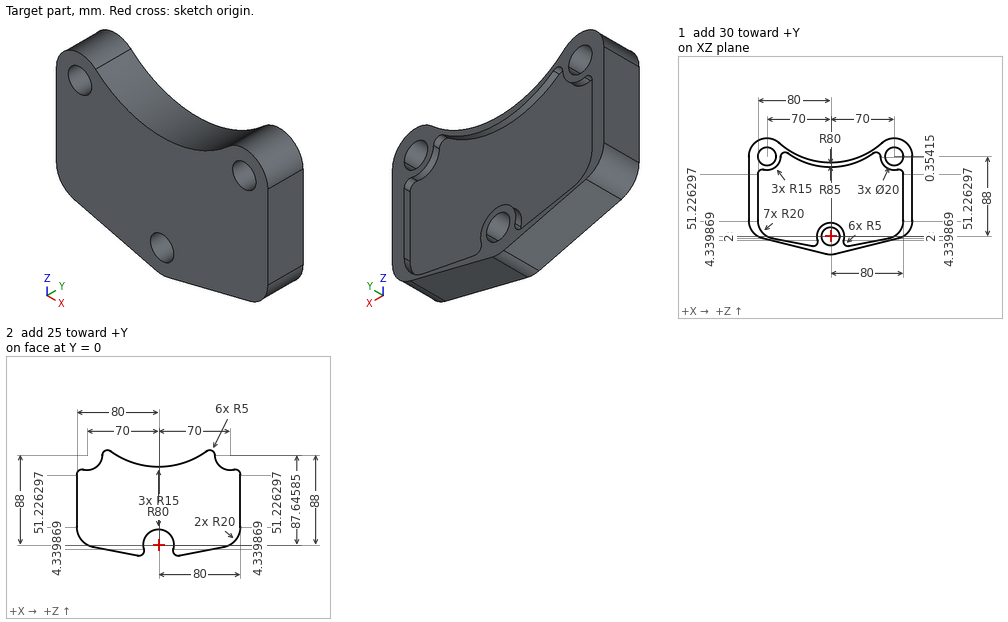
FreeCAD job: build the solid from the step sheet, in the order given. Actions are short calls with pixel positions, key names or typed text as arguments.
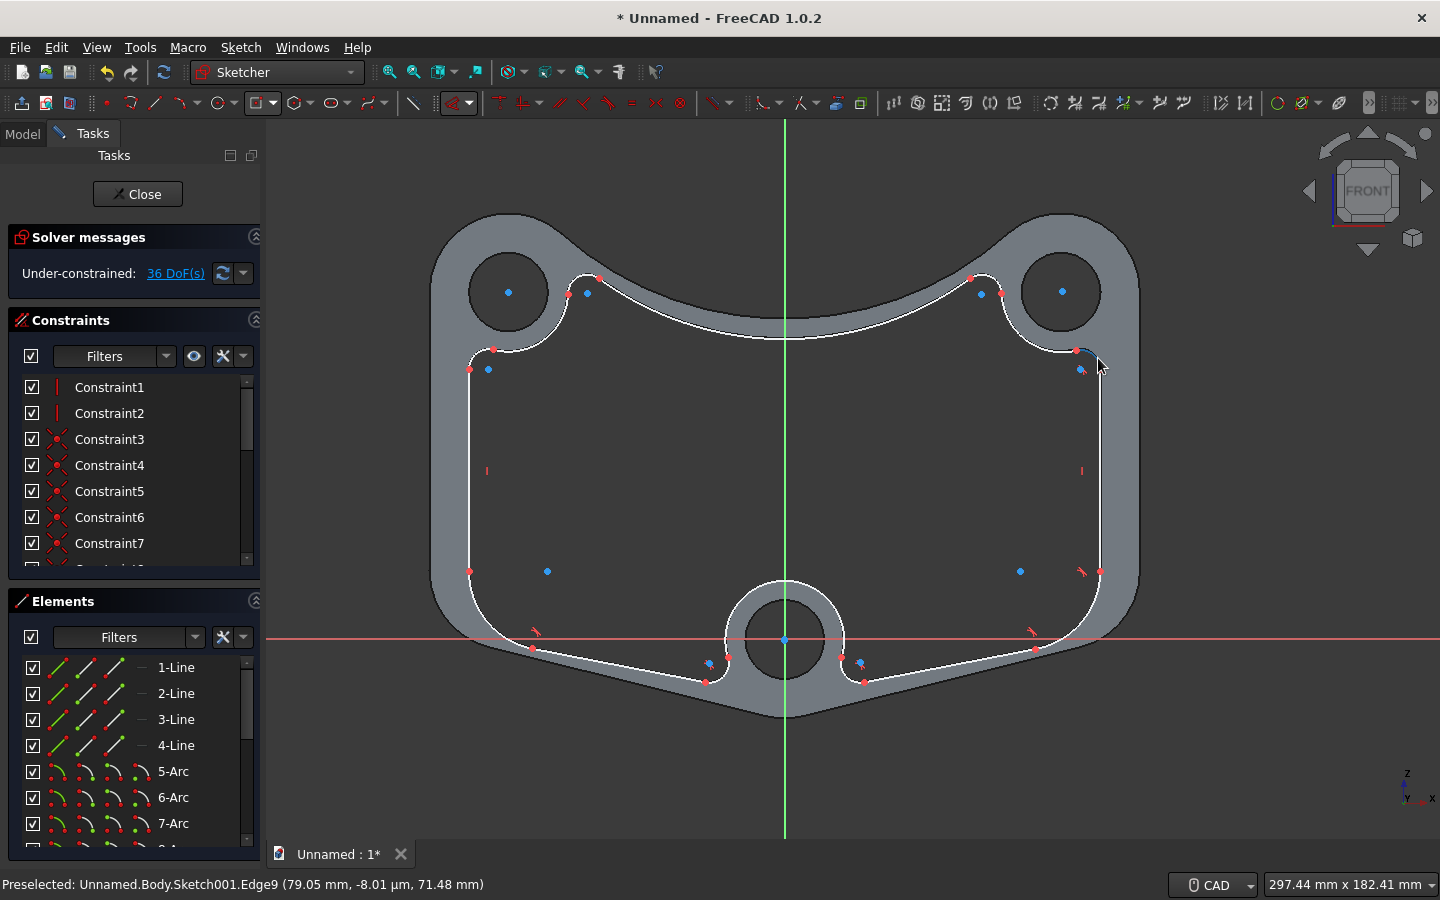
click(469, 430)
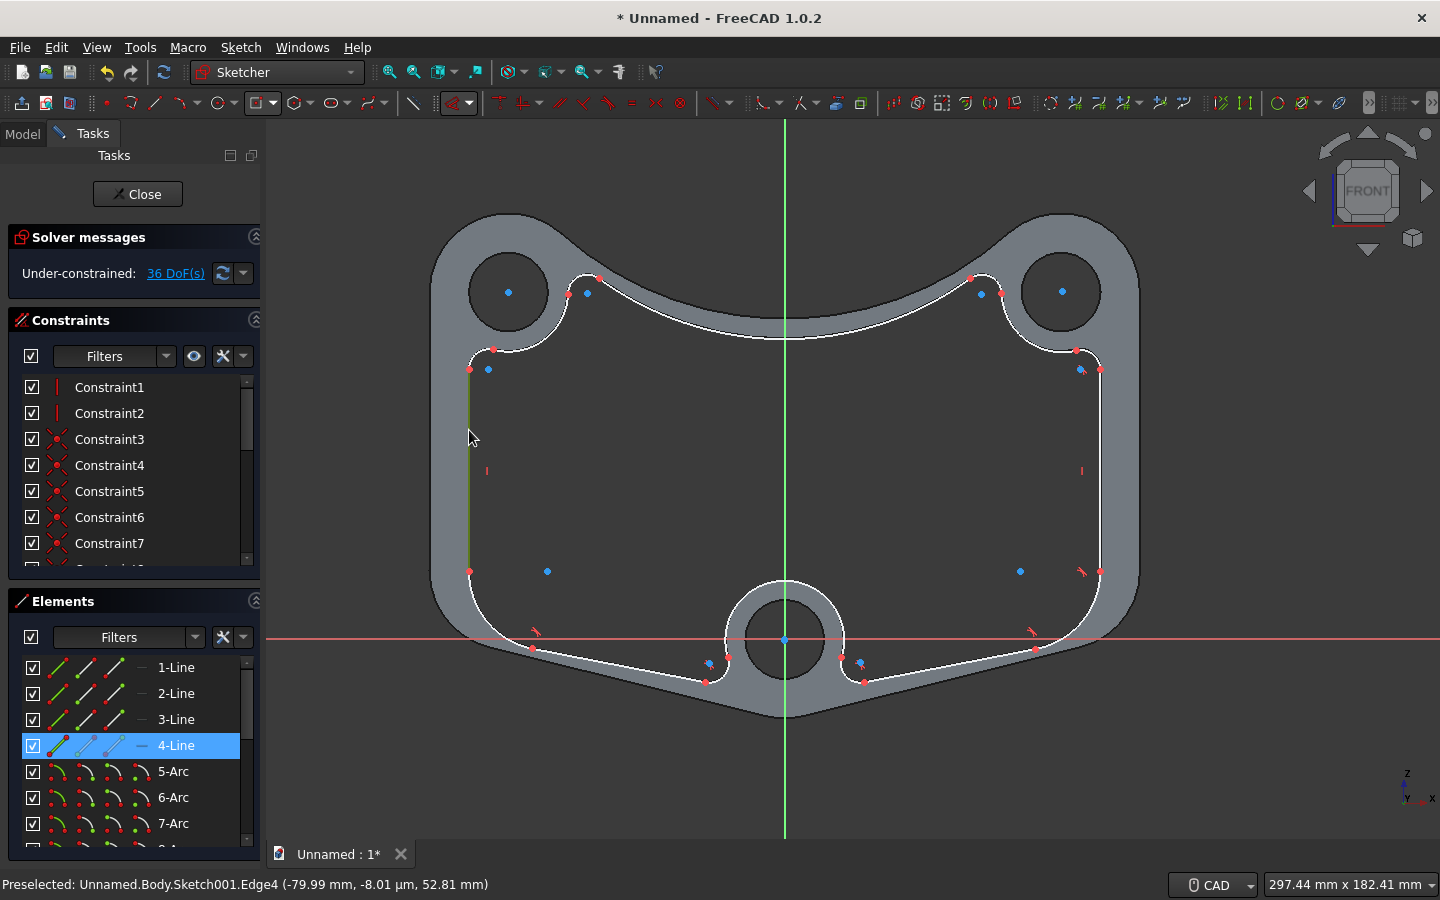
scroll(483, 350, up, 2)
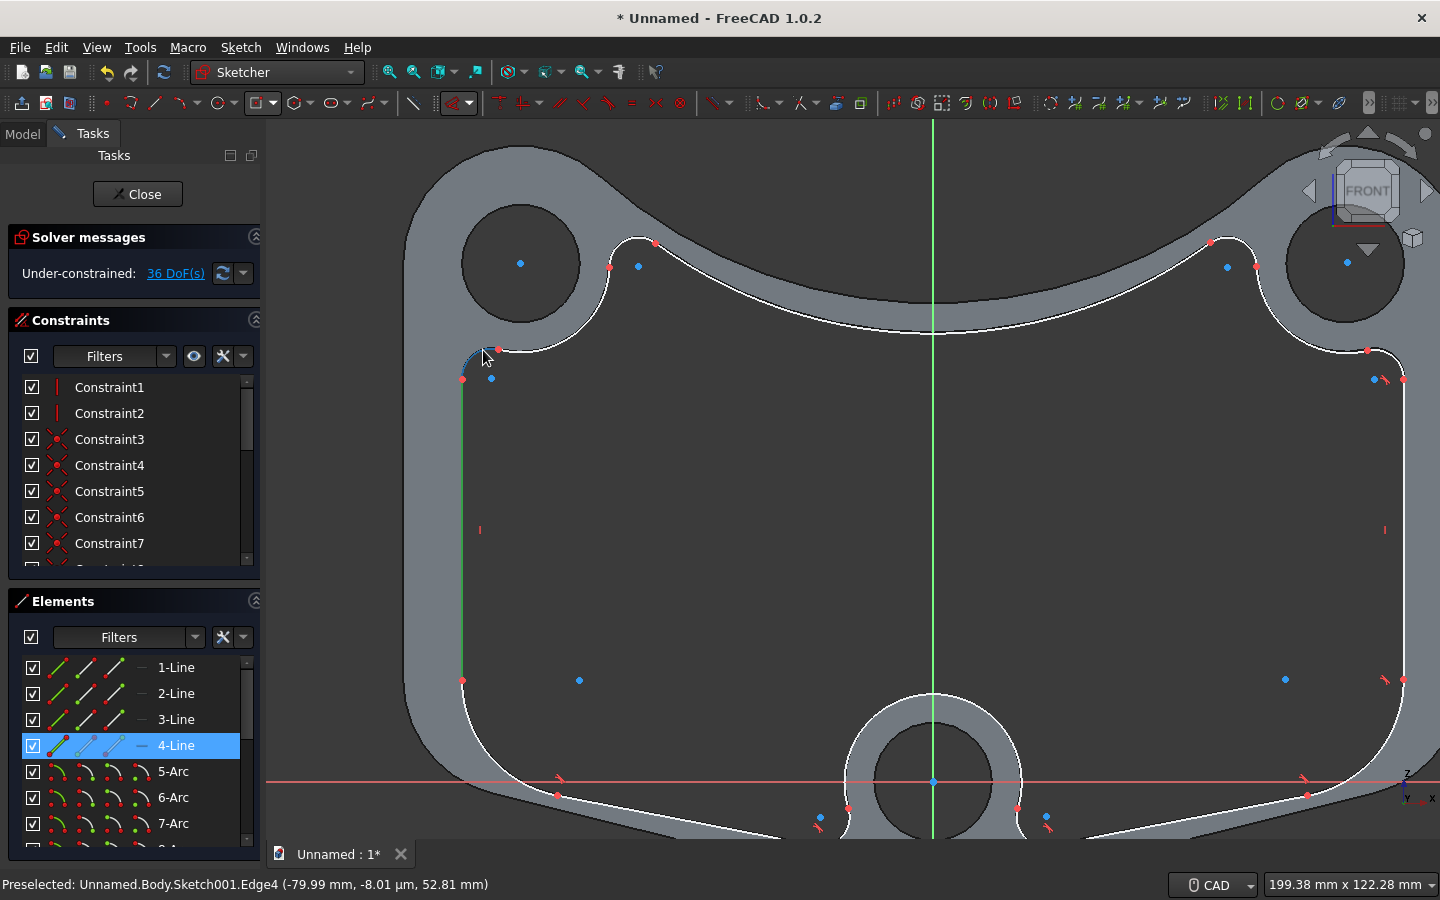
click(483, 350)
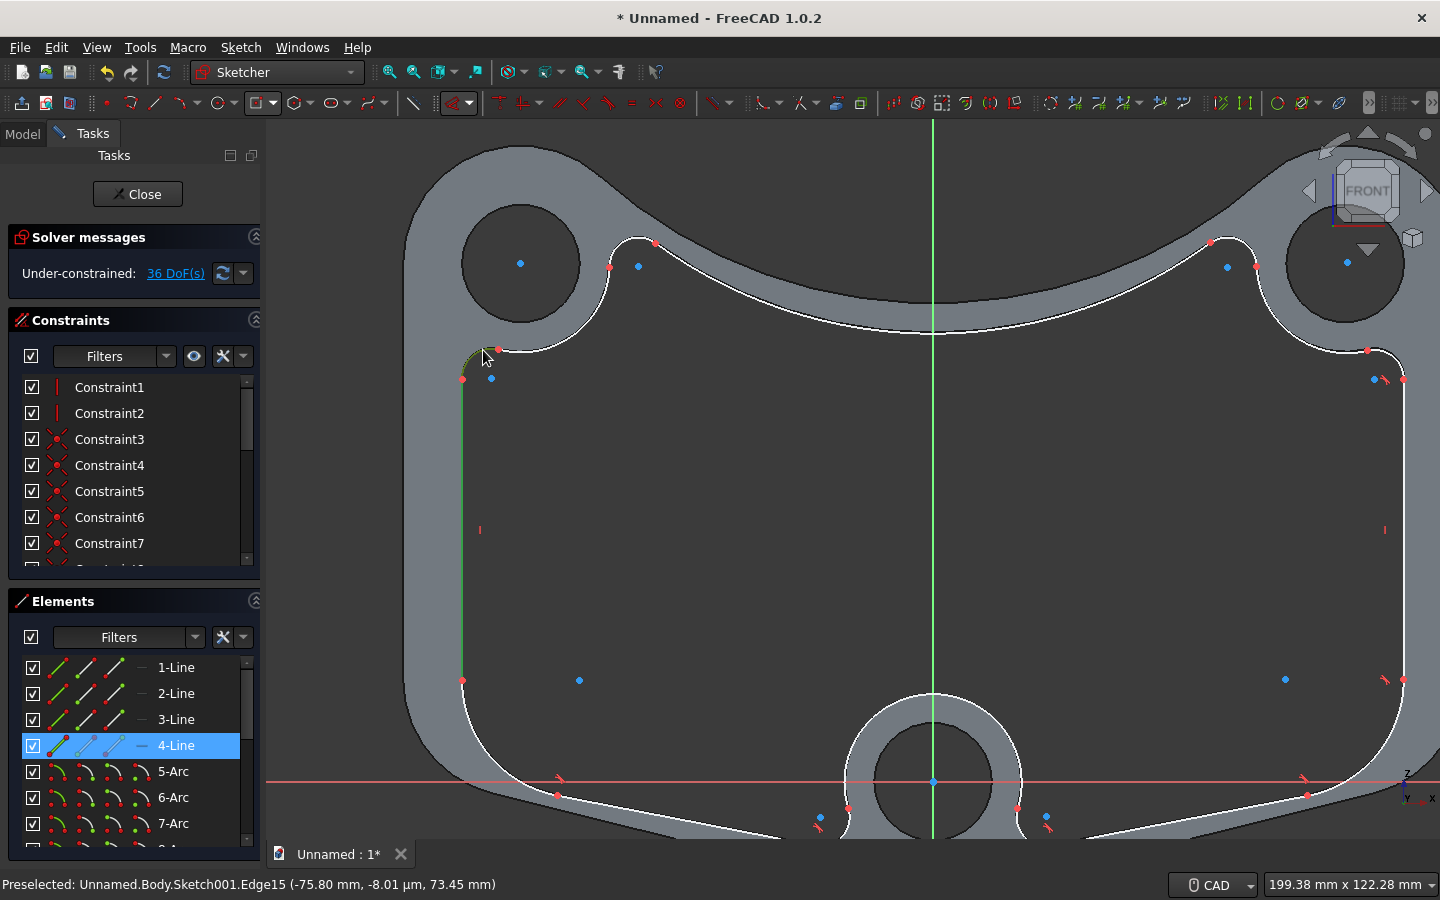
key(t)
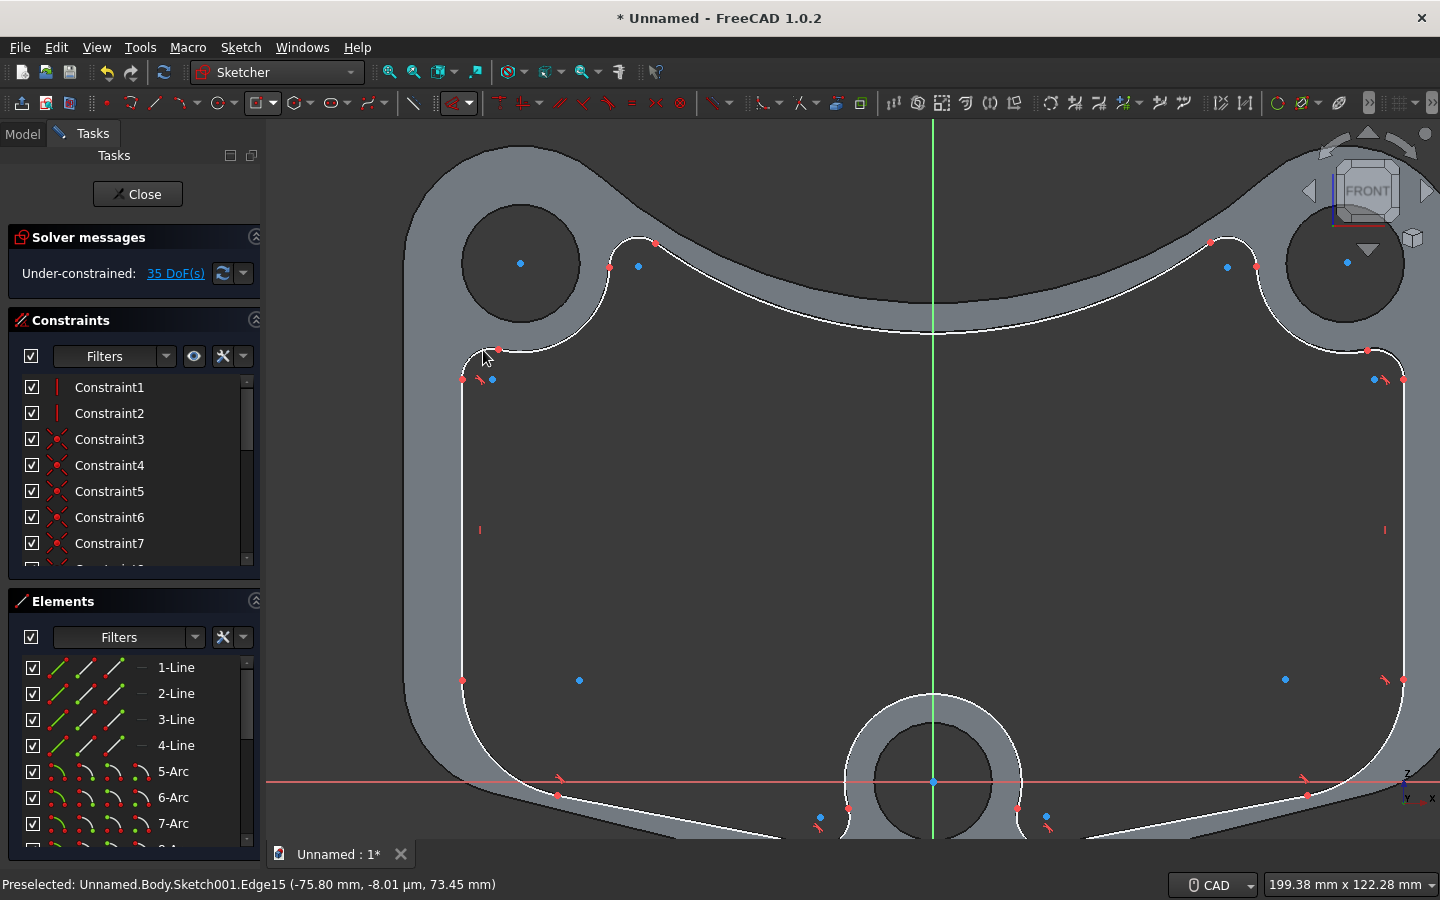
click(462, 470)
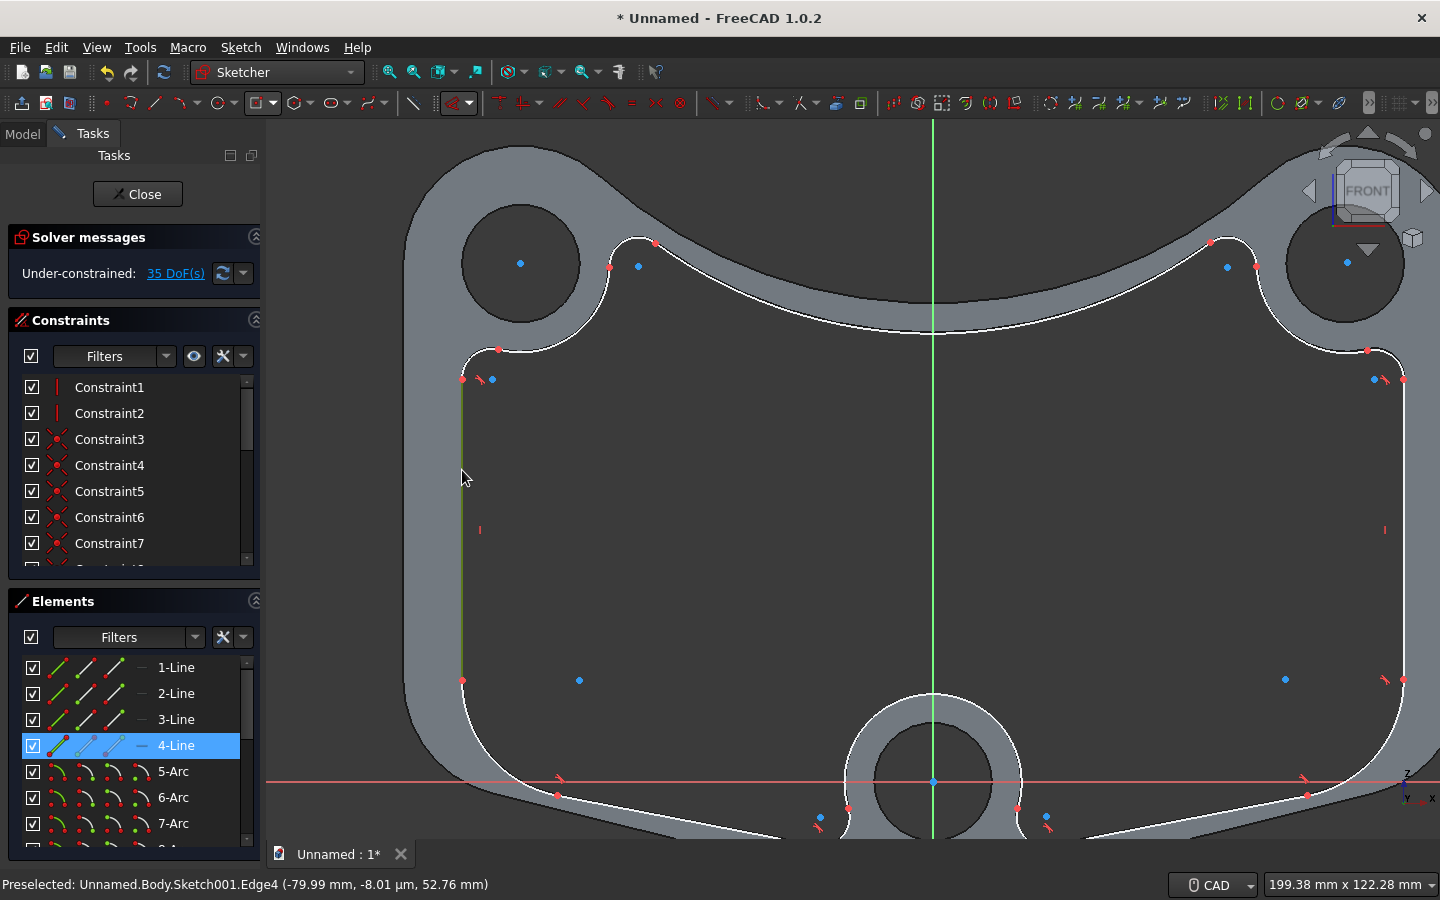
click(472, 728)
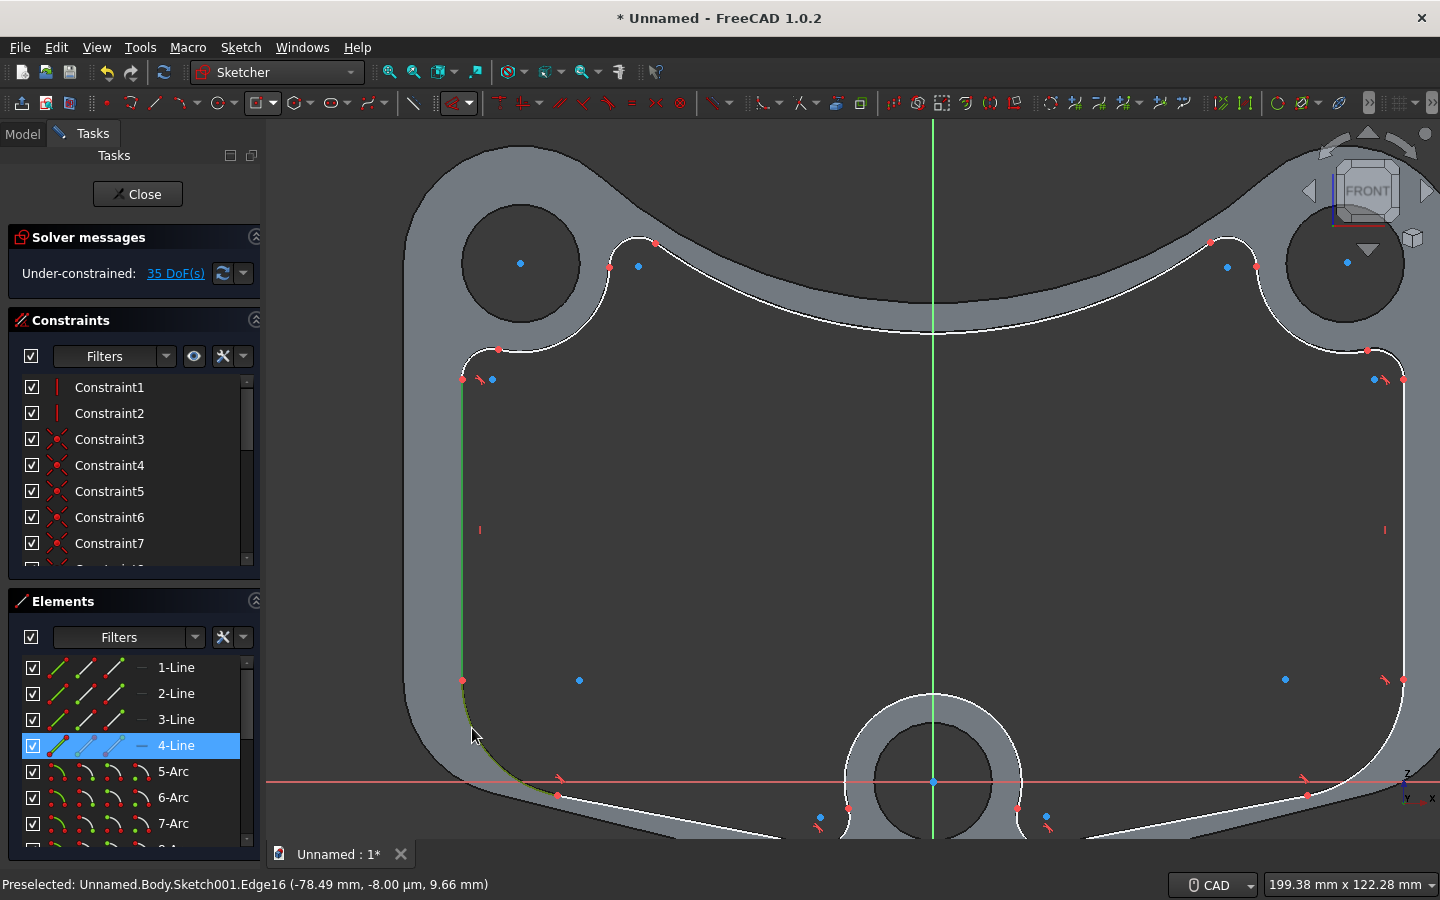
click(608, 104)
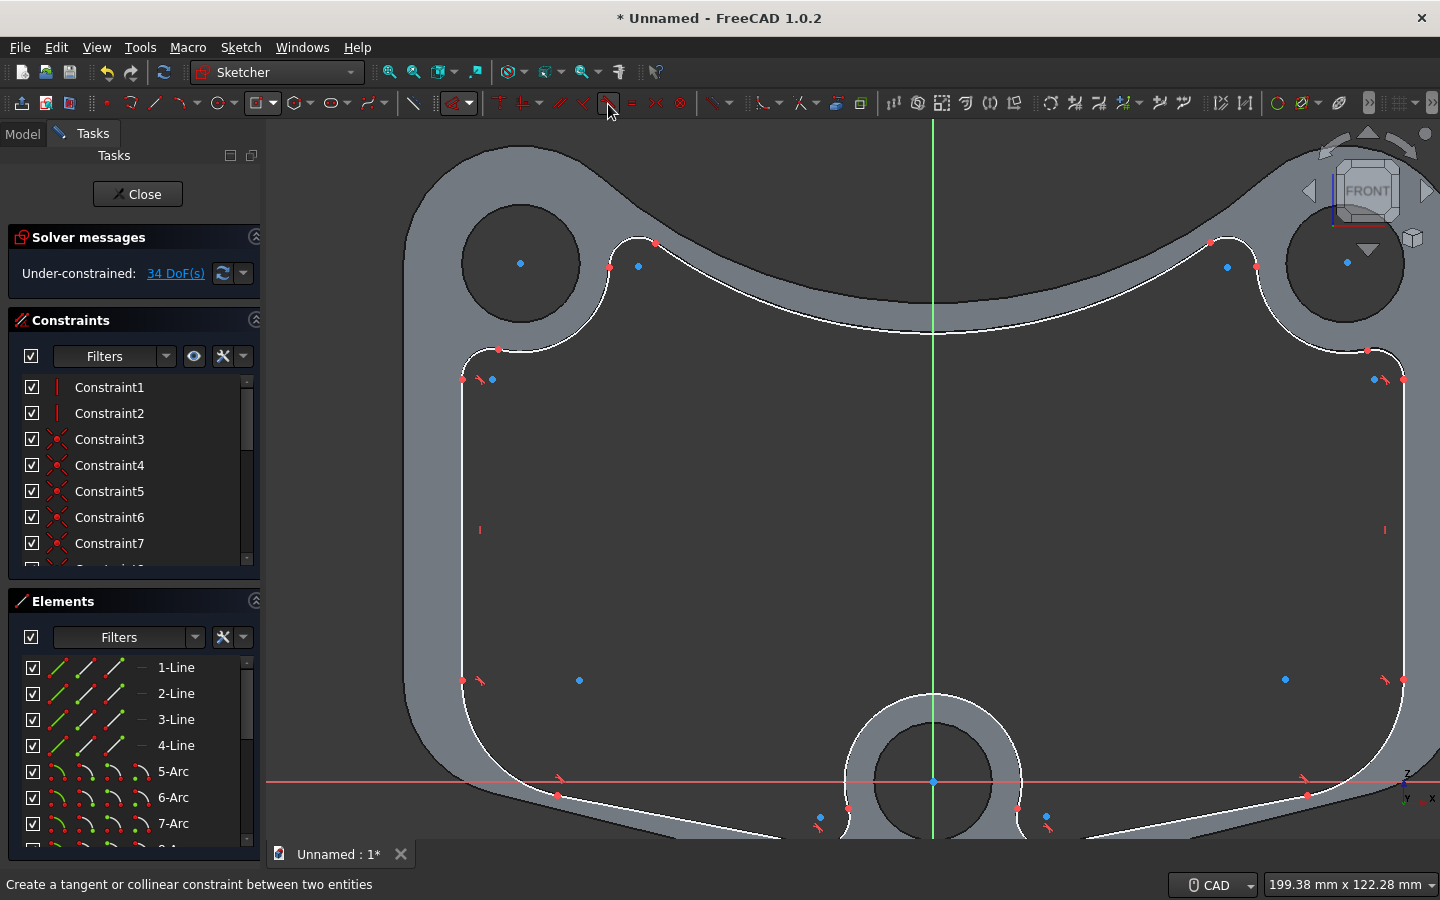
scroll(482, 350, down, 2)